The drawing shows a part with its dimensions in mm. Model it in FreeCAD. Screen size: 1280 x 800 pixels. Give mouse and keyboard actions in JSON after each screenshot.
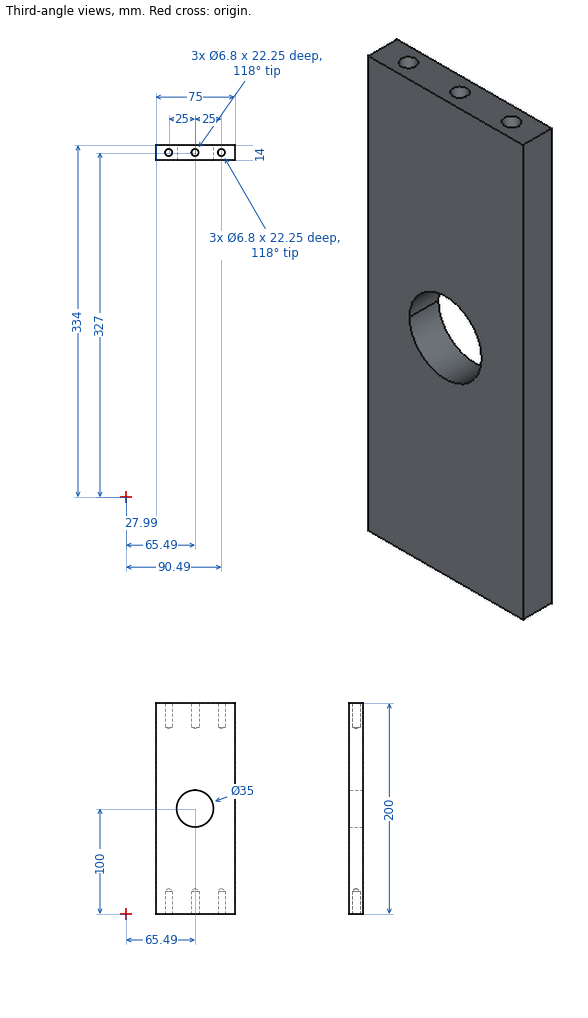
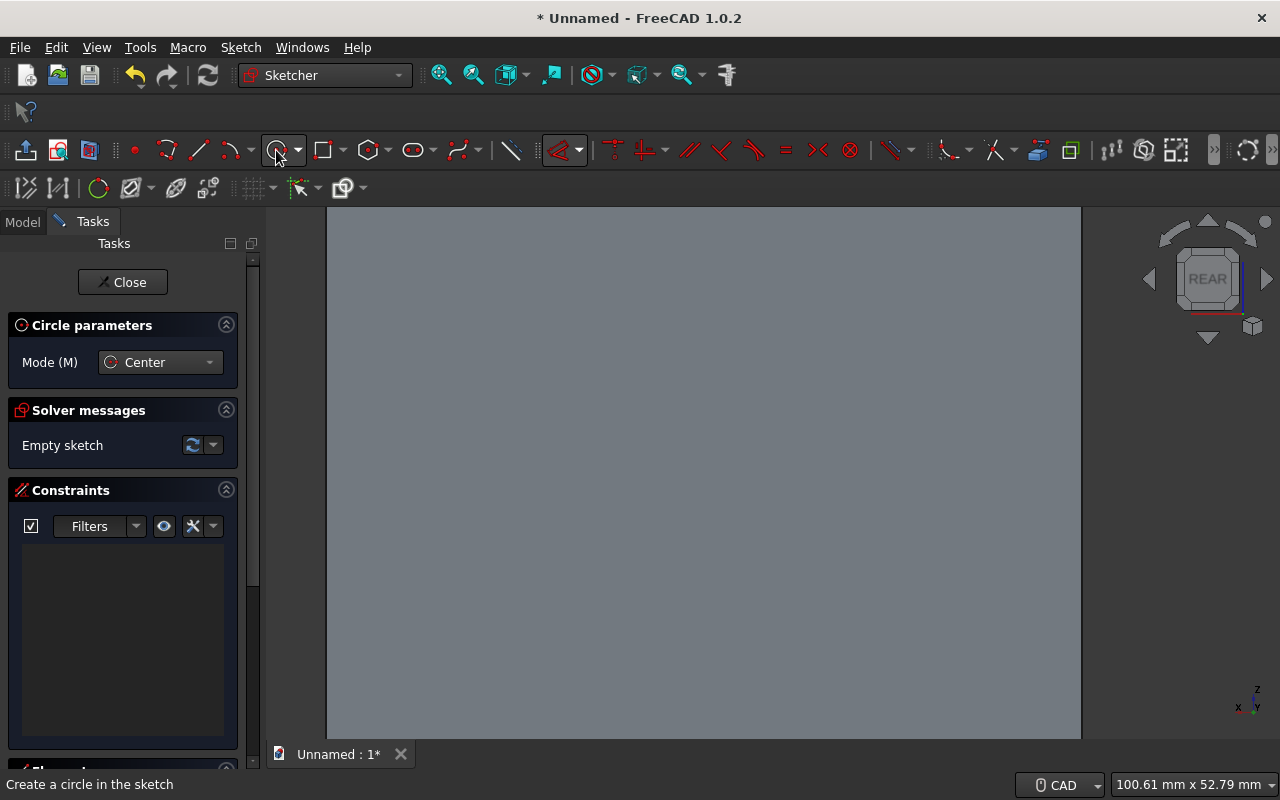
{"action": "left_click", "coordinate": [704, 471]}
{"action": "mouse_move", "coordinate": [829, 347]}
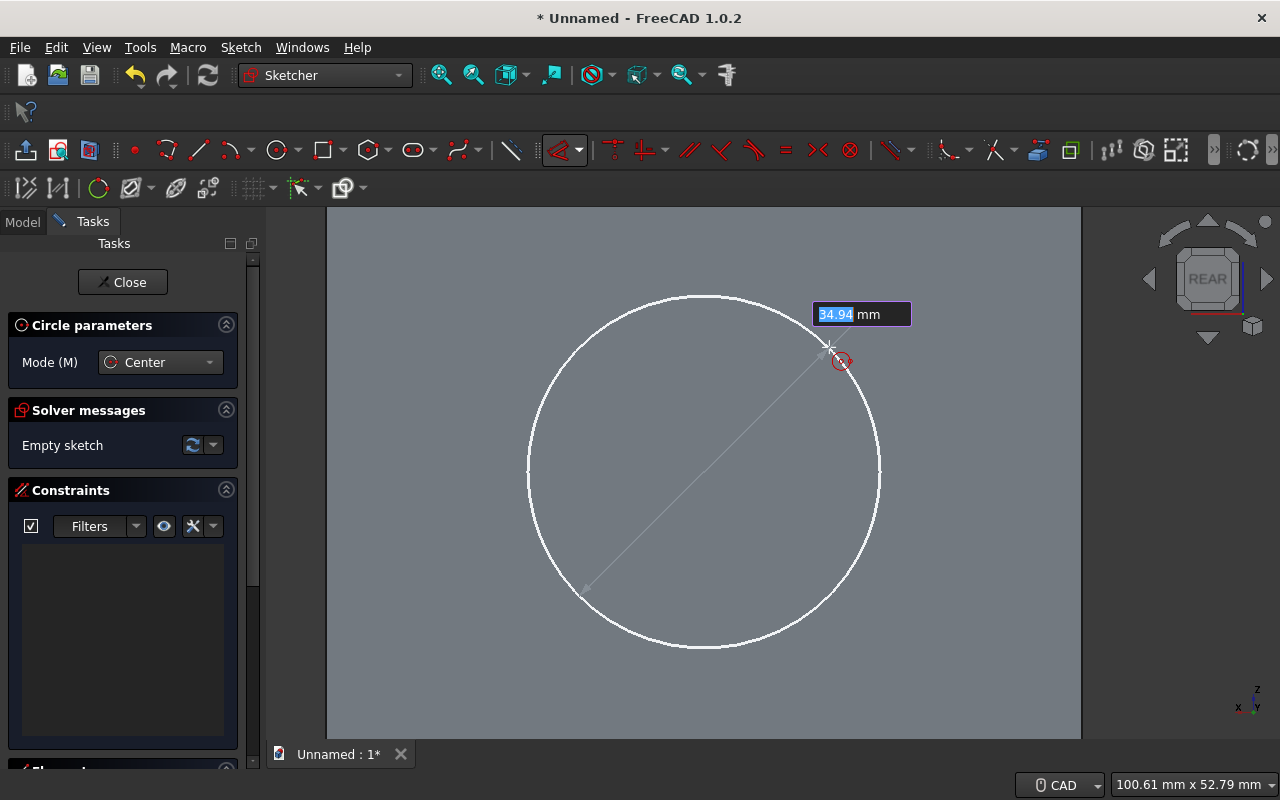
{"action": "type", "text": "35"}
{"action": "key", "text": "Return"}
{"action": "key", "text": "Escape"}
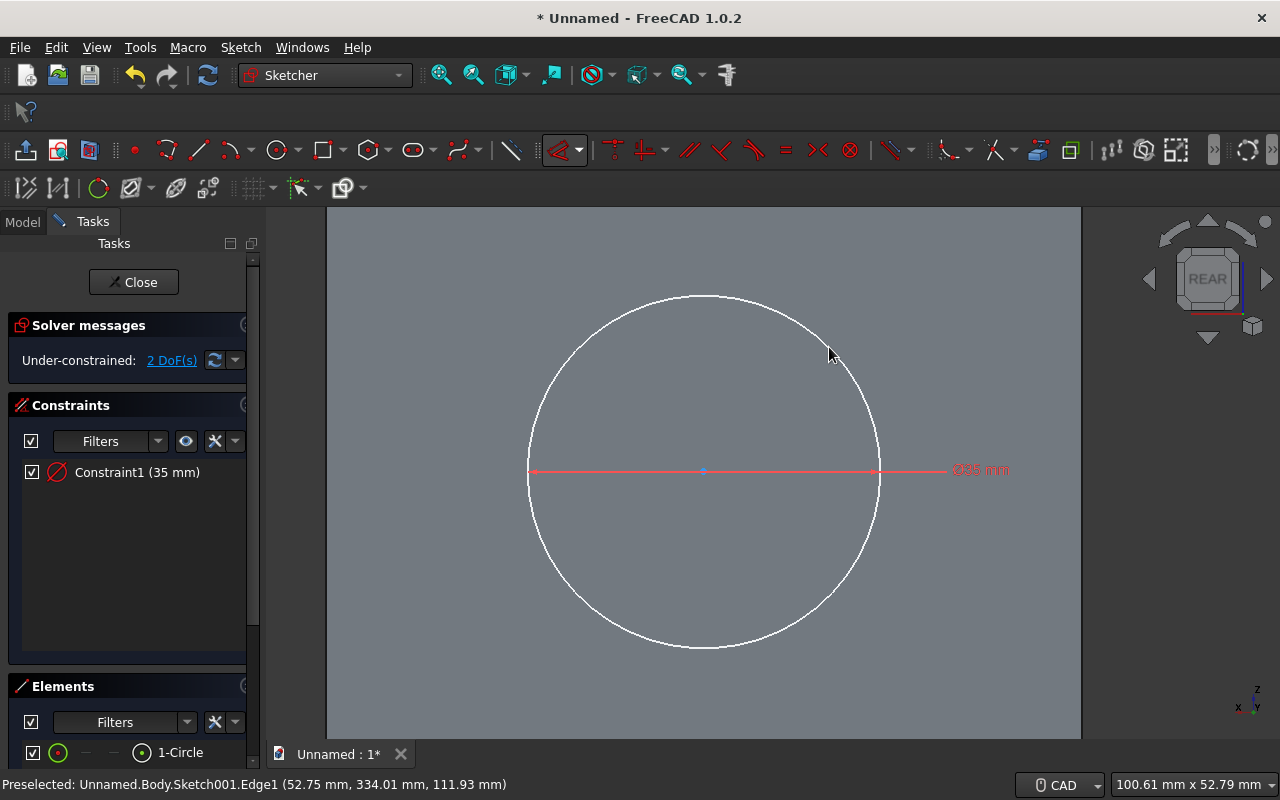
{"action": "left_click", "coordinate": [704, 472]}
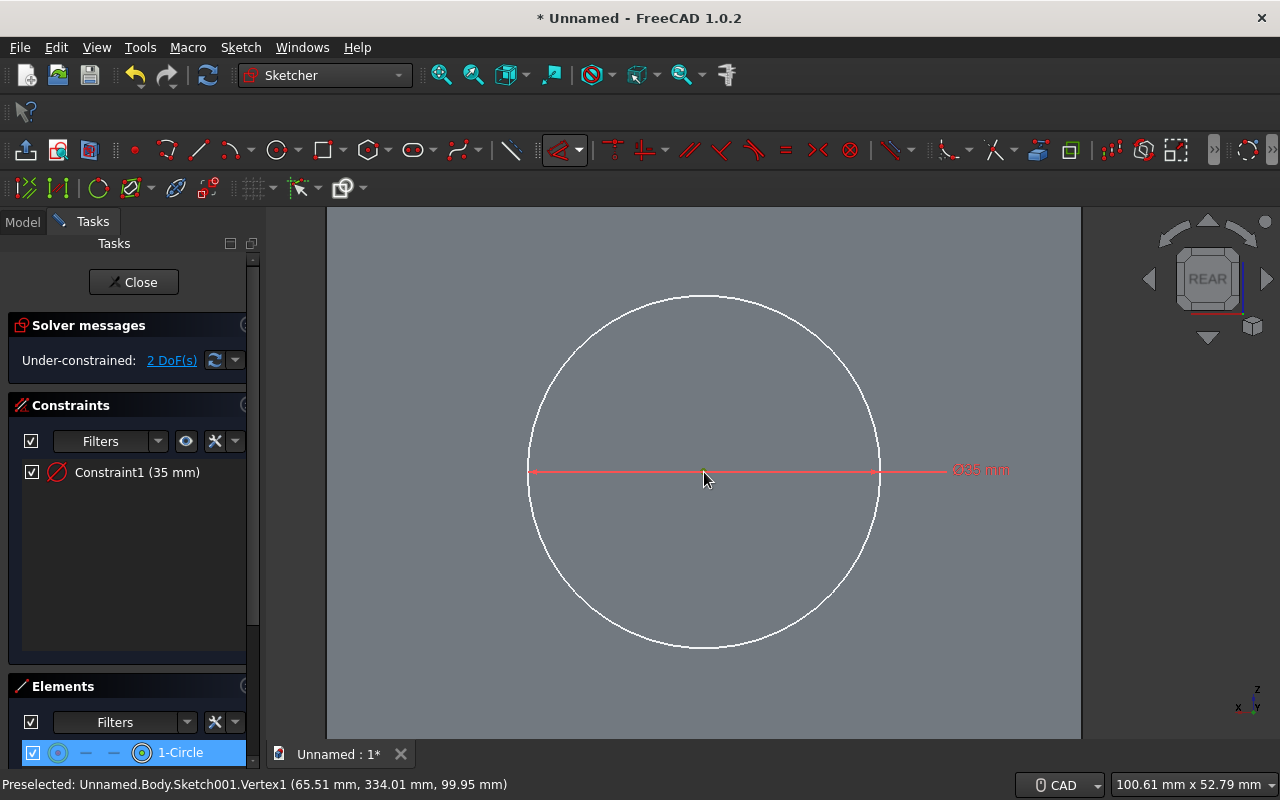
{"action": "left_click", "coordinate": [582, 150]}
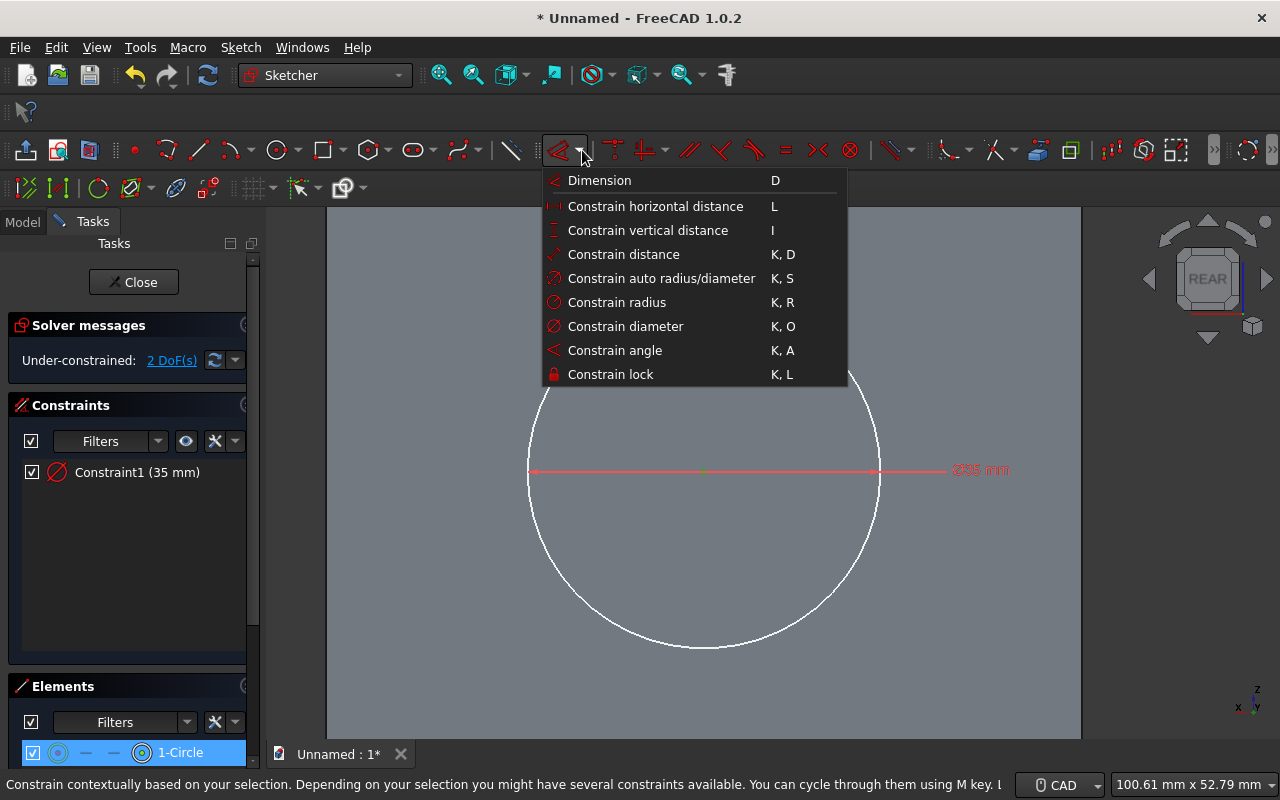
{"action": "left_click", "coordinate": [695, 230]}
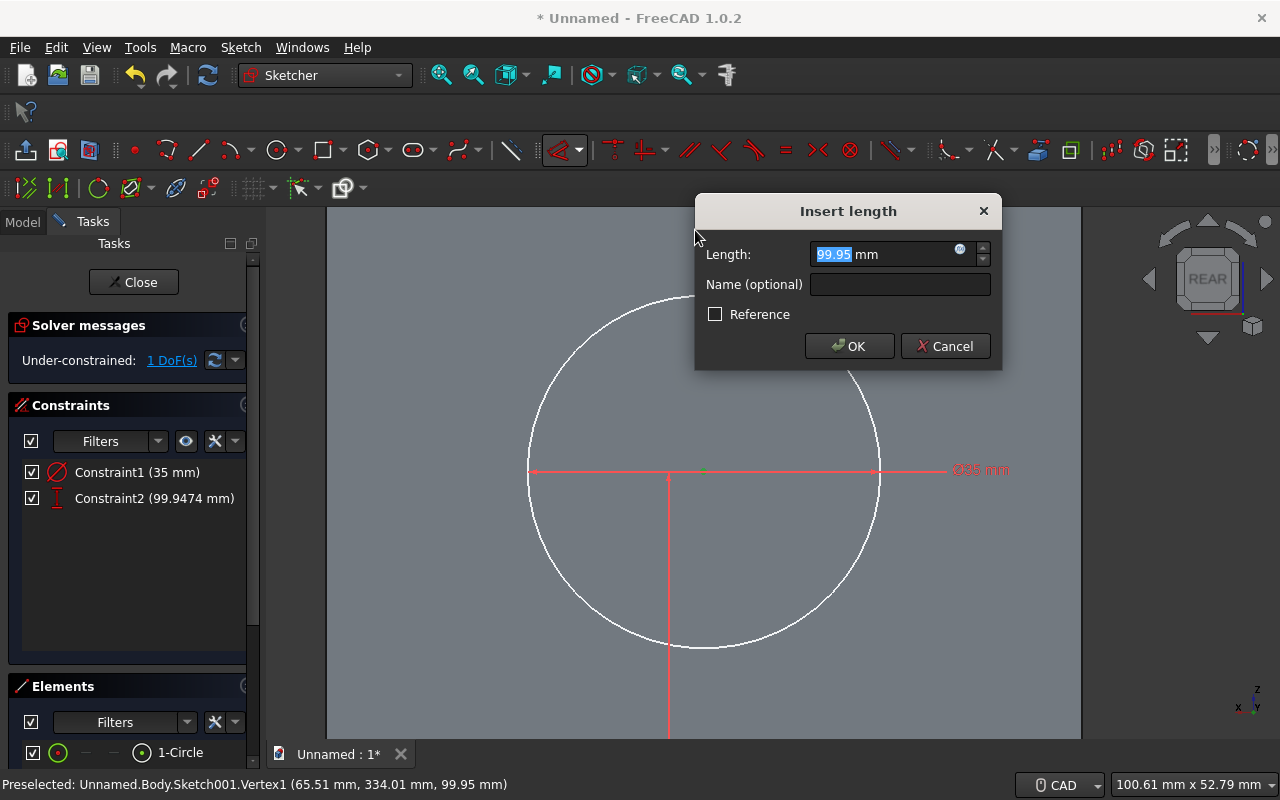
{"action": "type", "text": "100"}
{"action": "key", "text": "Return"}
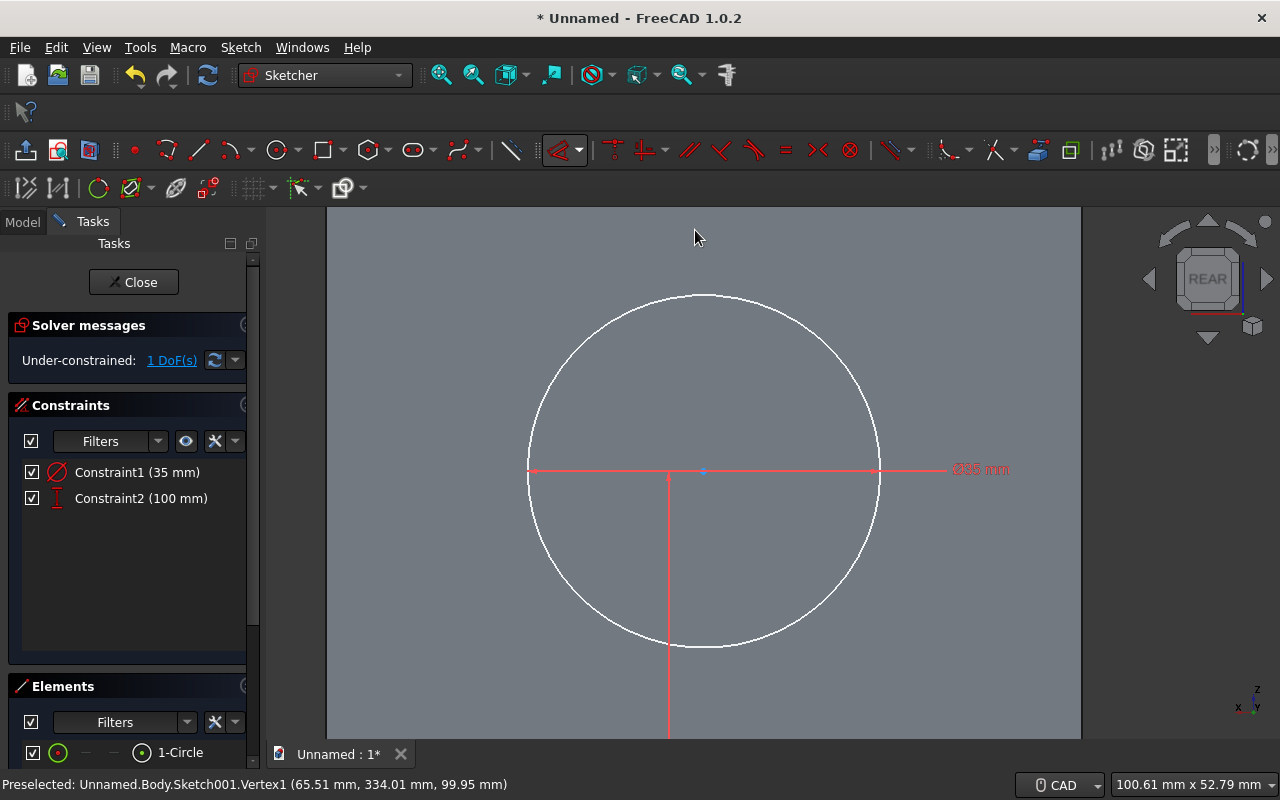
{"action": "left_click", "coordinate": [704, 471]}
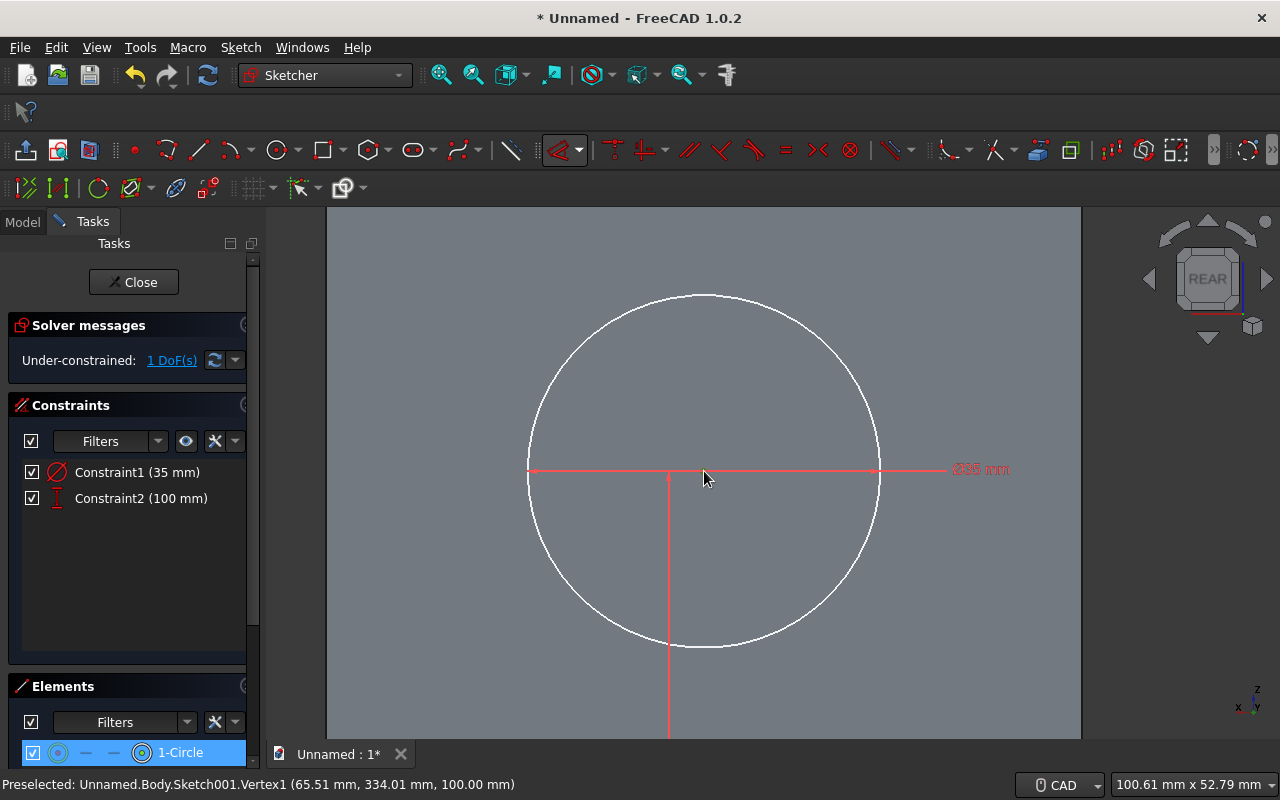
{"action": "left_click", "coordinate": [582, 150]}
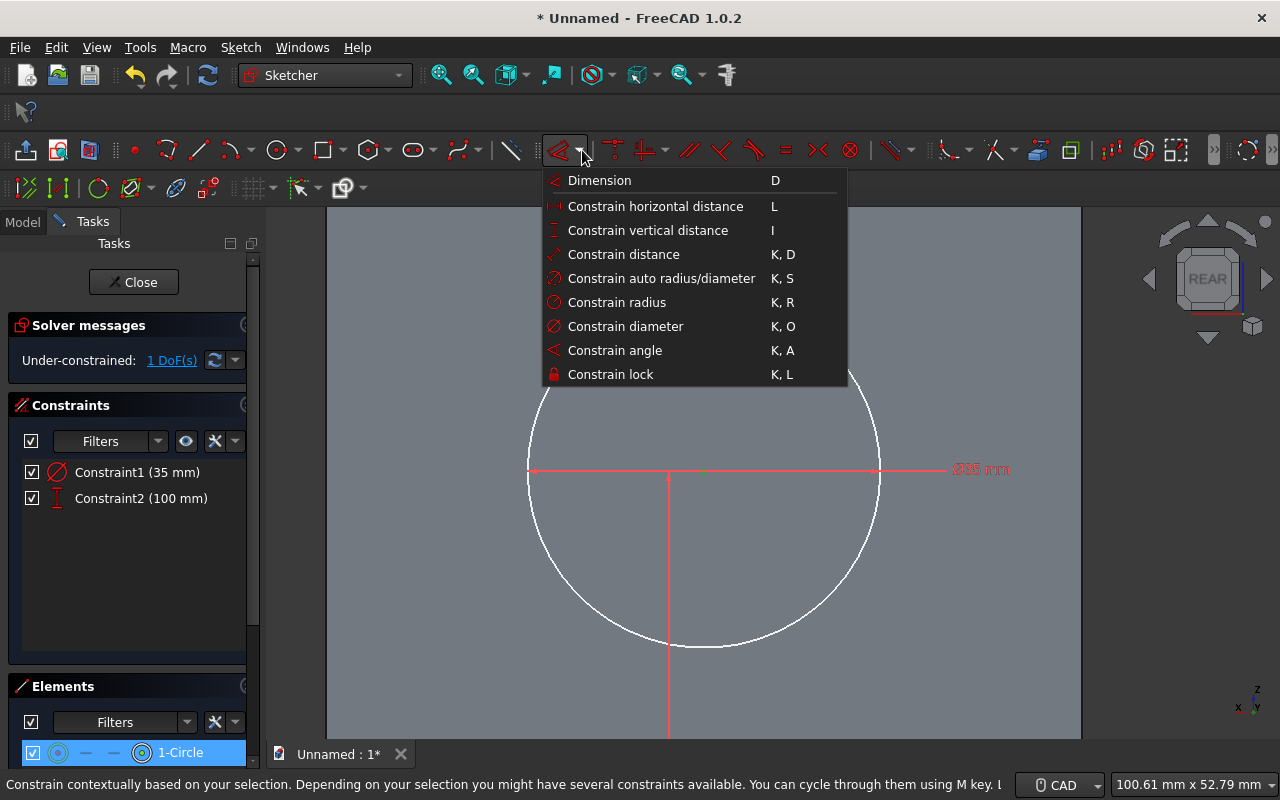
{"action": "left_click", "coordinate": [695, 206]}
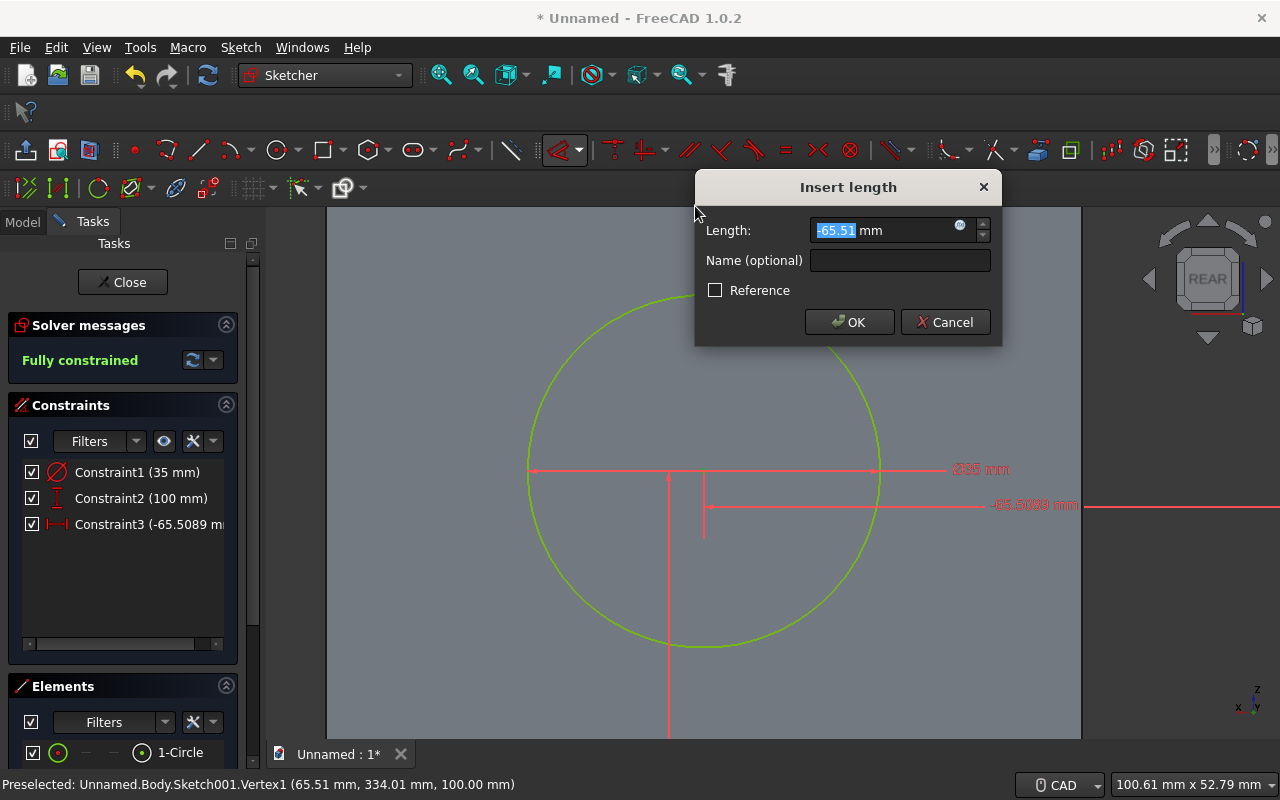
{"action": "type", "text": "-65.49"}
{"action": "key", "text": "Return"}